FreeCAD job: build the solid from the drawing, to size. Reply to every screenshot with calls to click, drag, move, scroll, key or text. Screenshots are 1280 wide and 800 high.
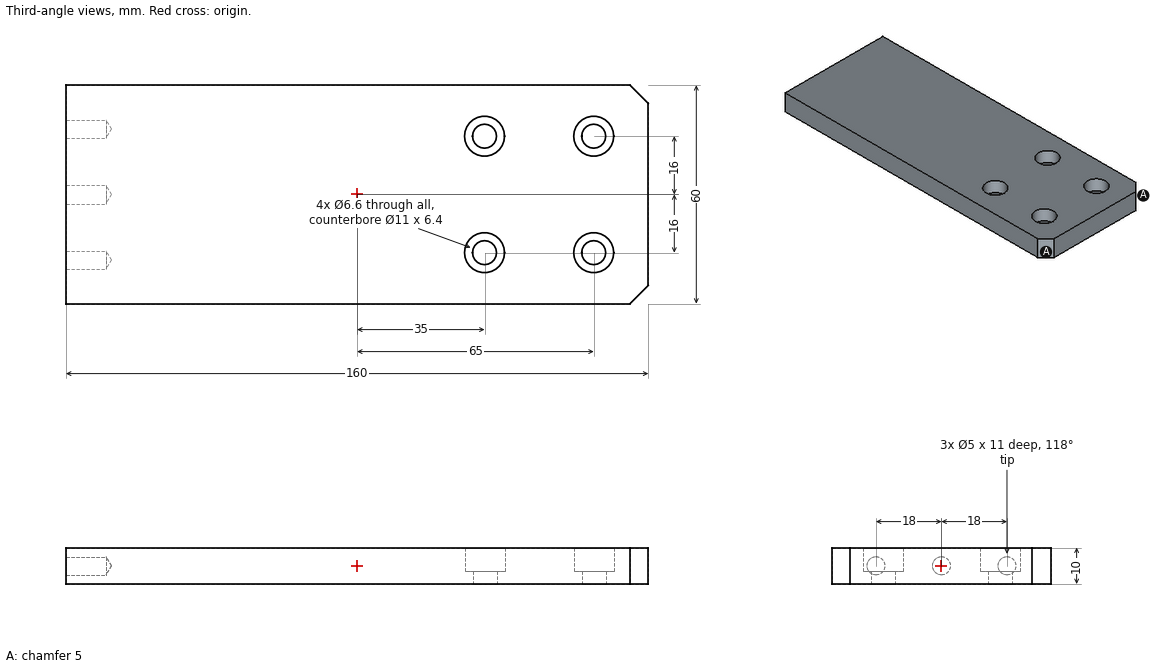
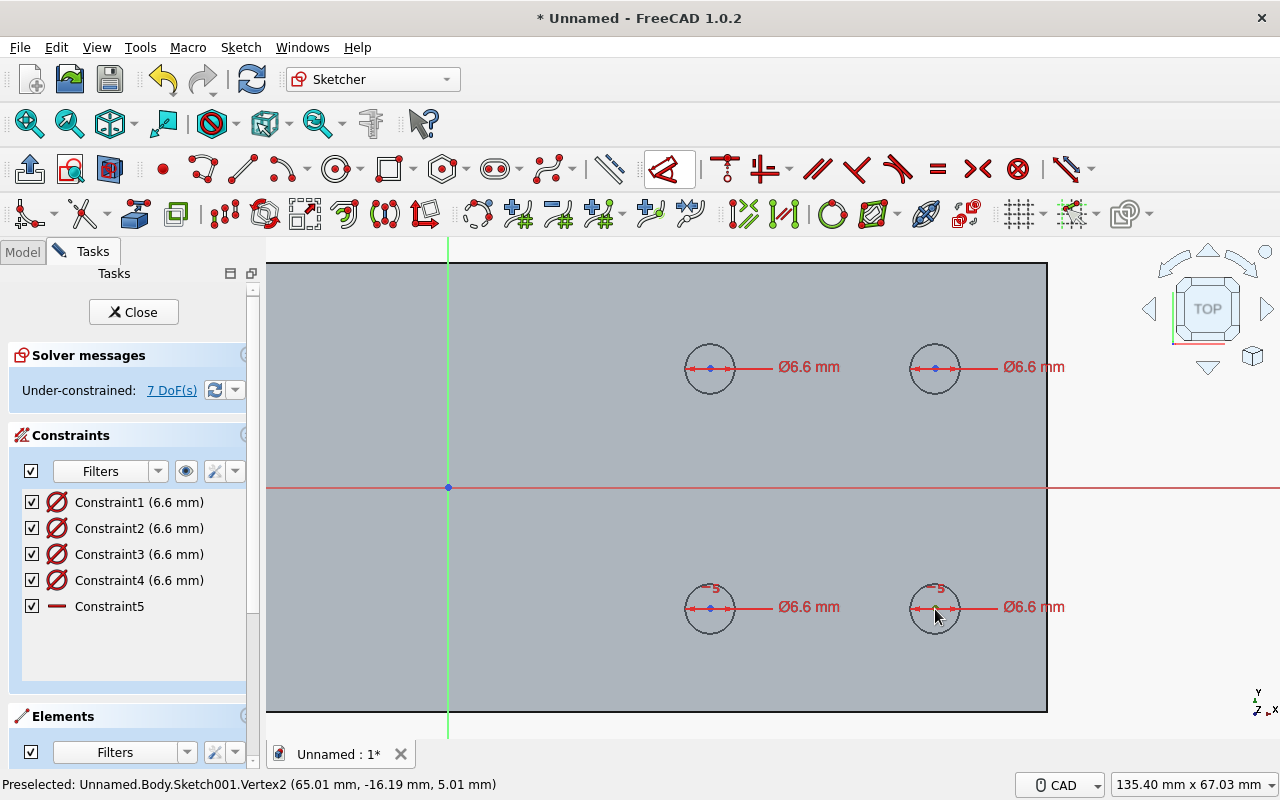
click(935, 369)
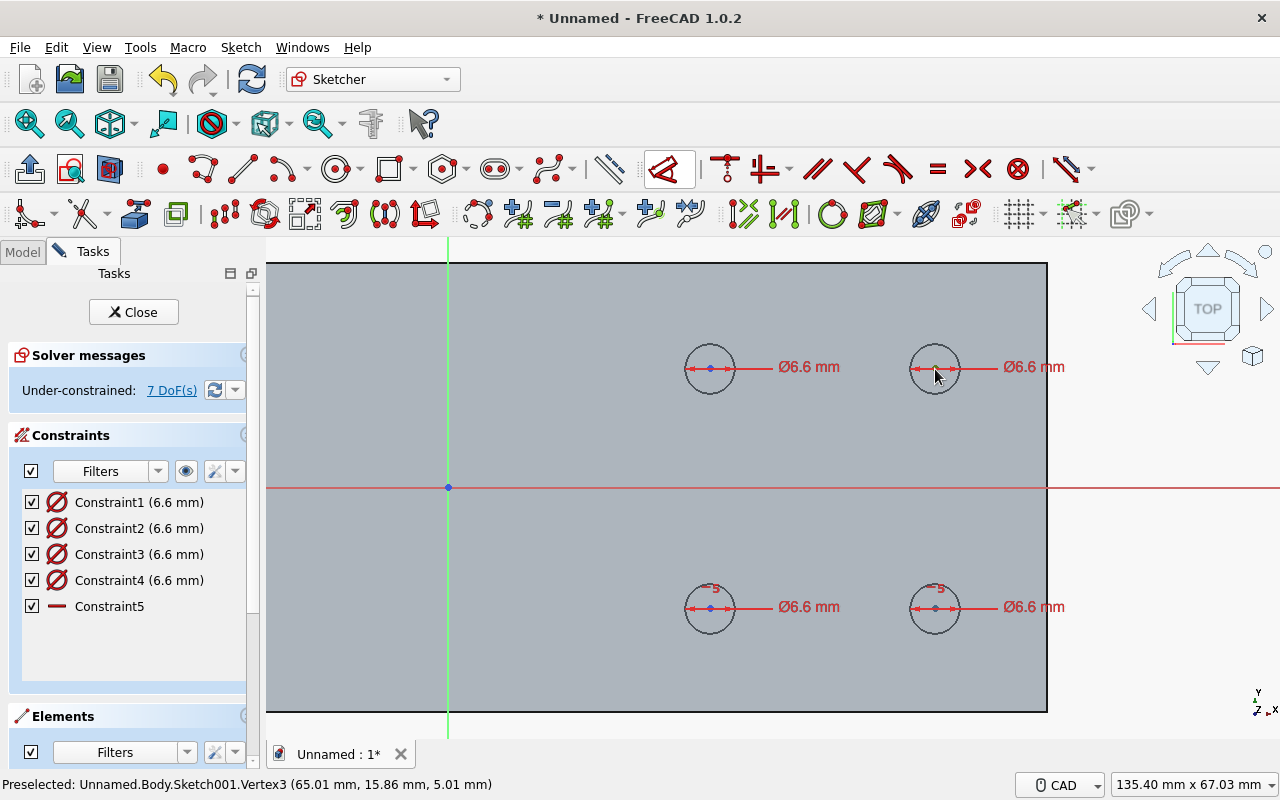
key(v)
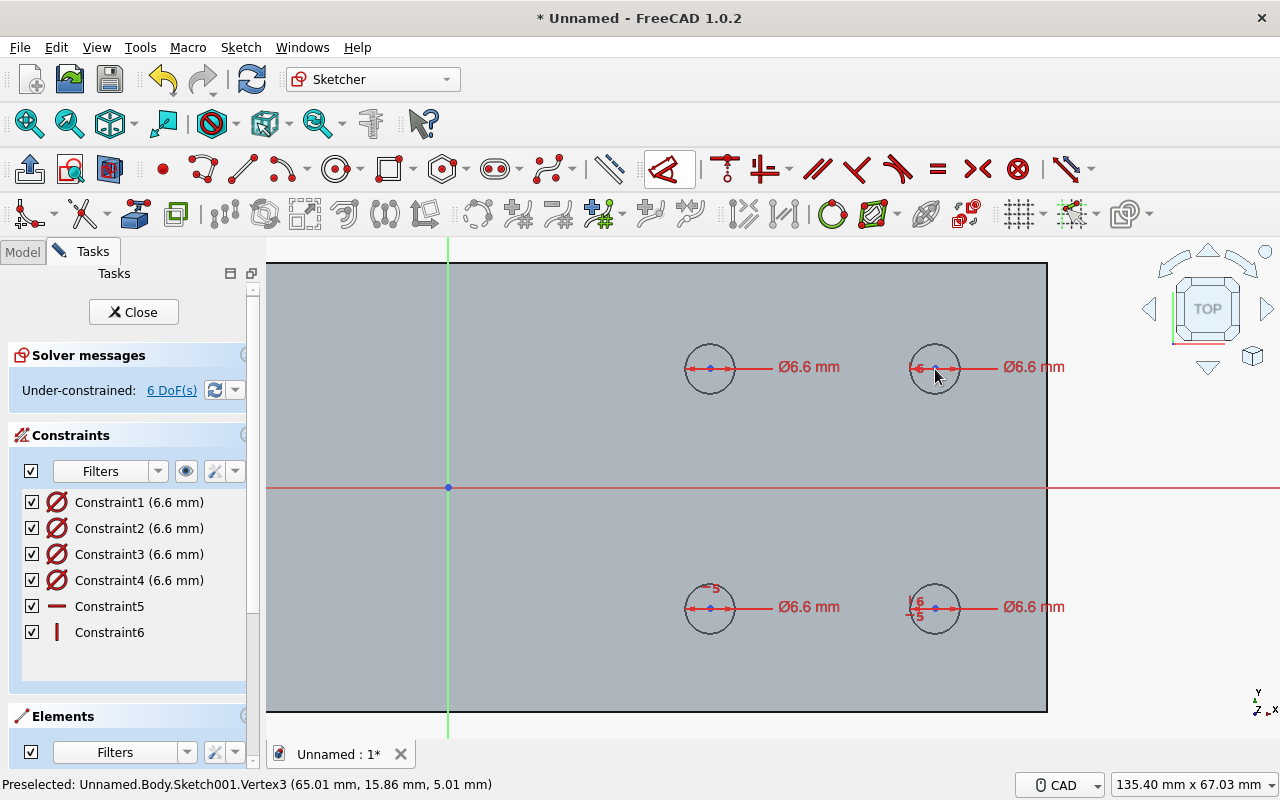
click(710, 609)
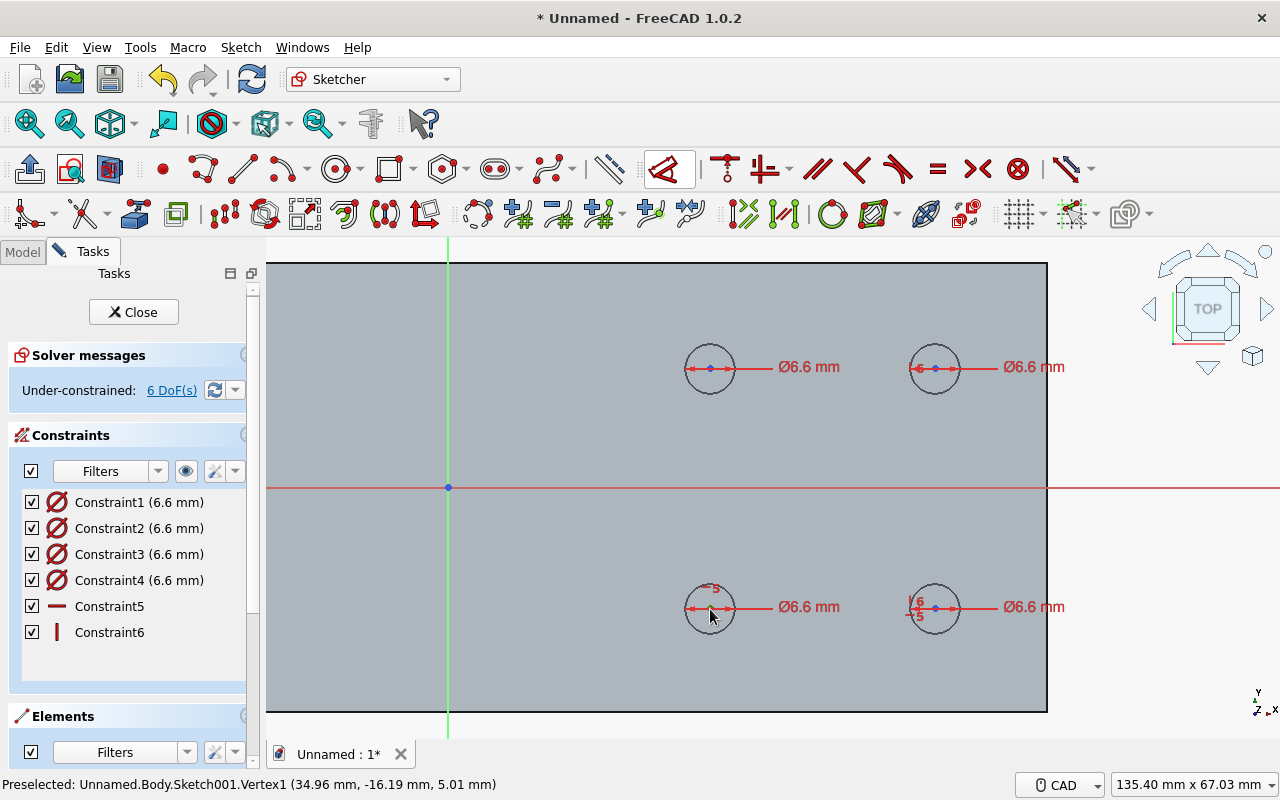
click(710, 369)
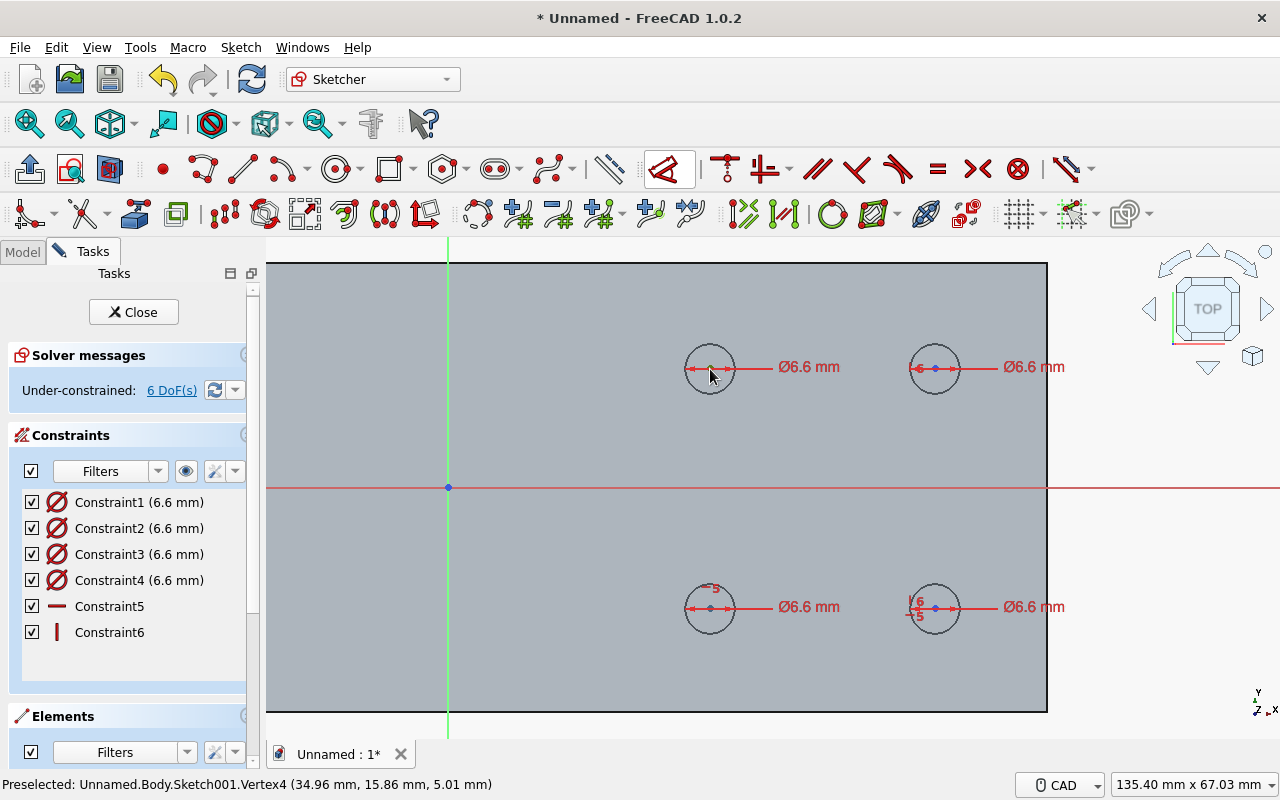
key(v)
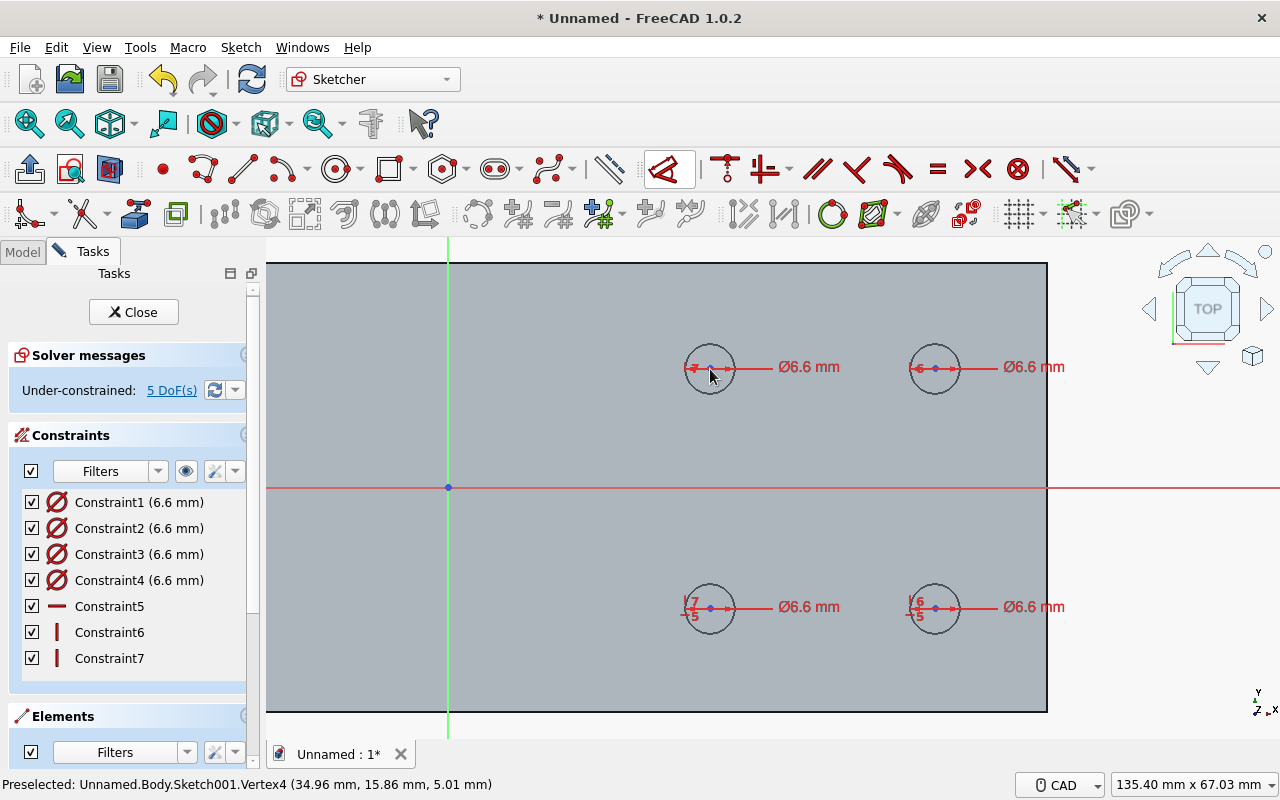
click(935, 369)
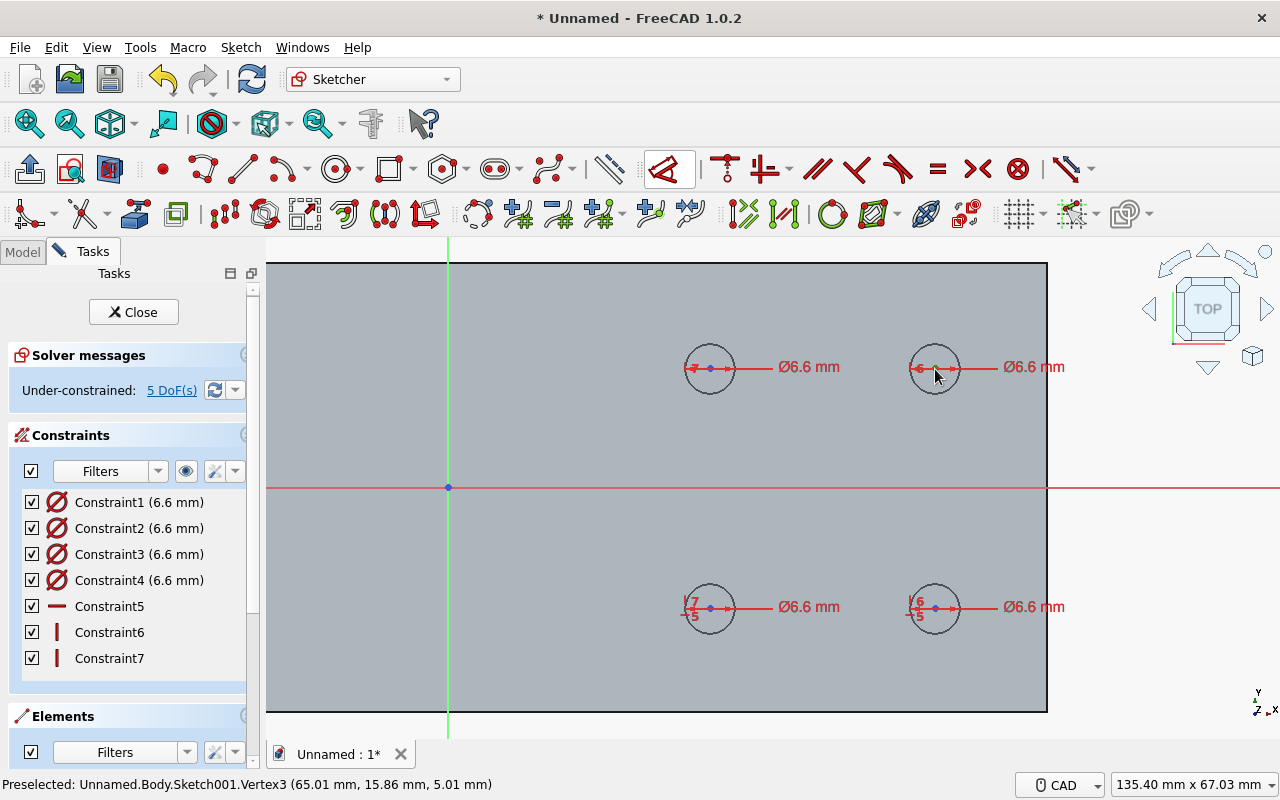
click(710, 369)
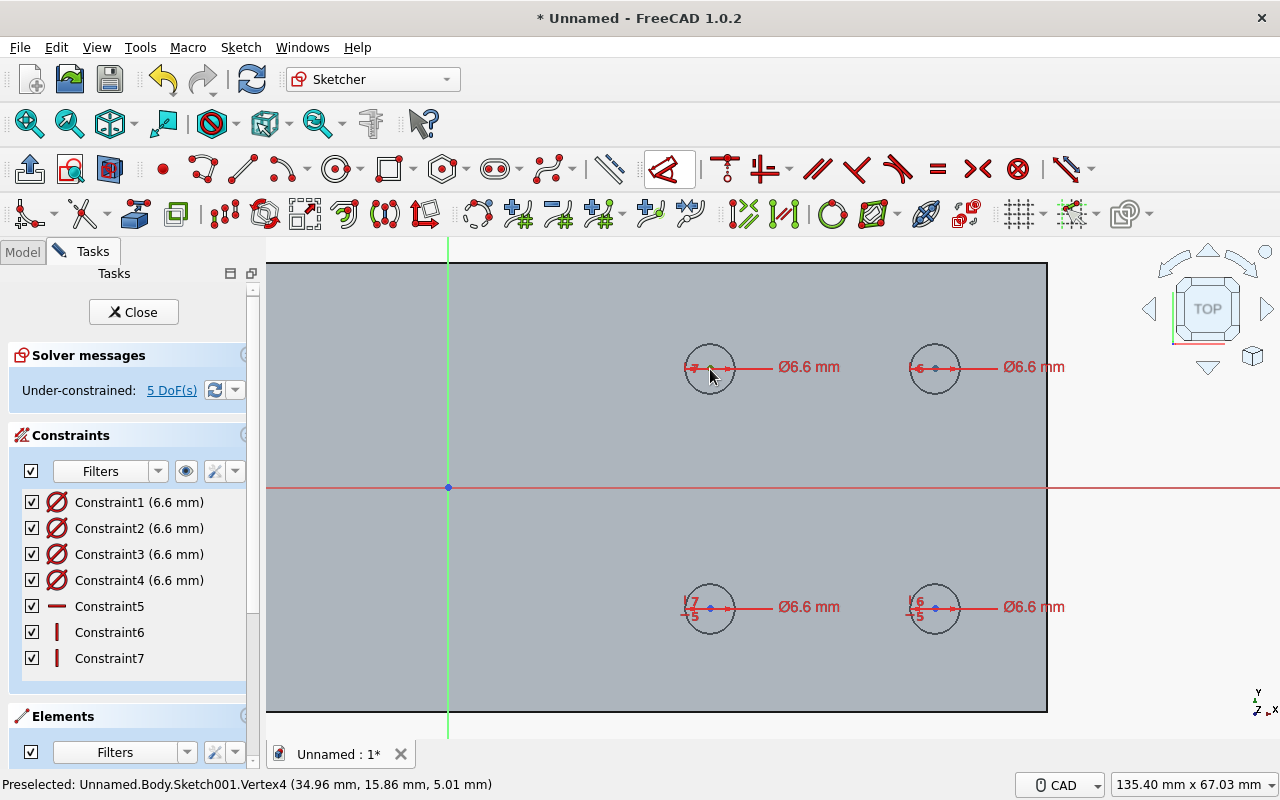
key(h)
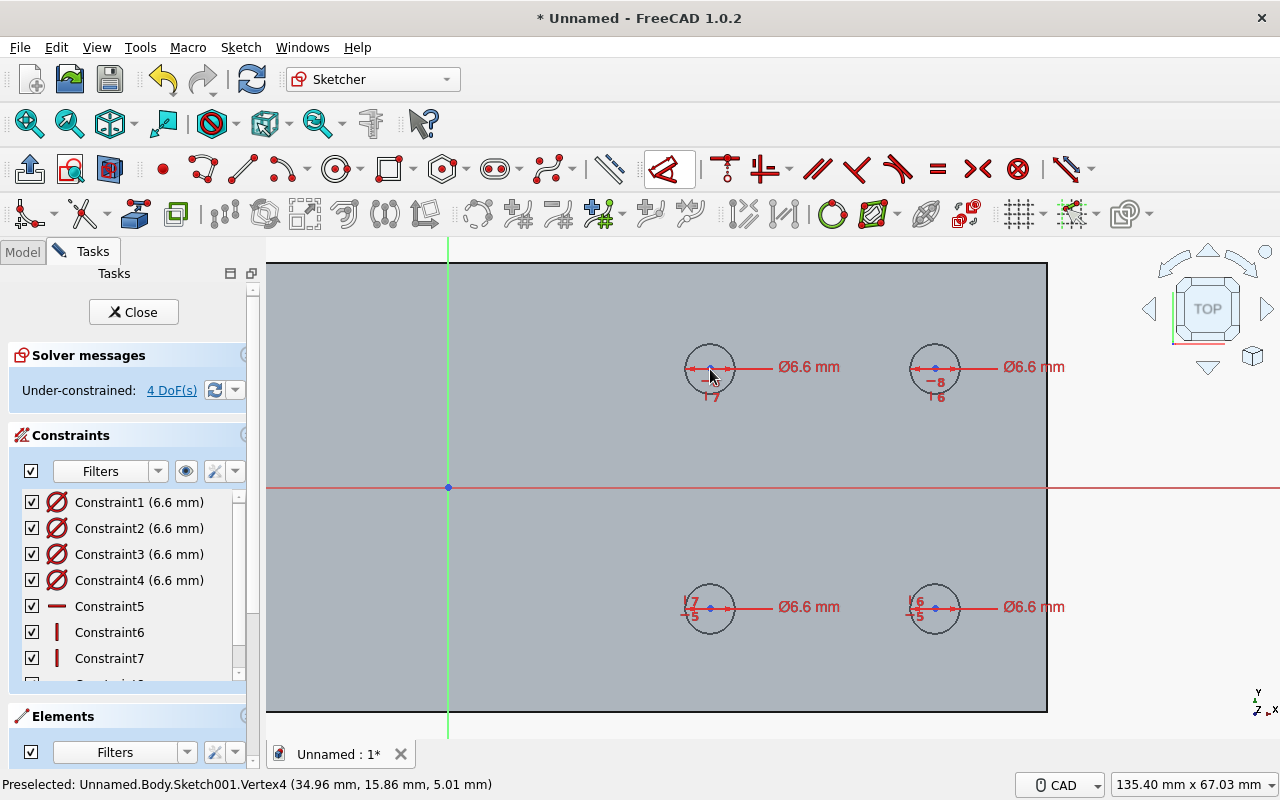
click(710, 609)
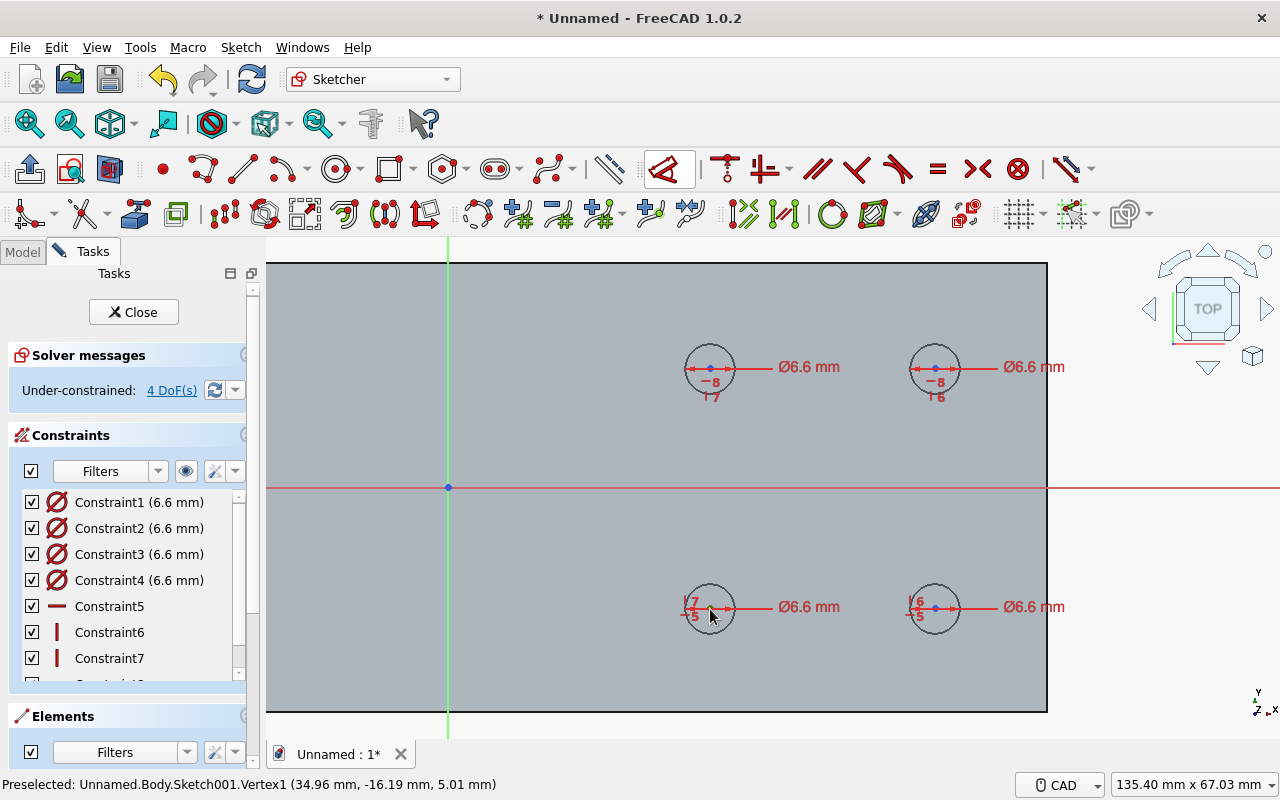
key(l)